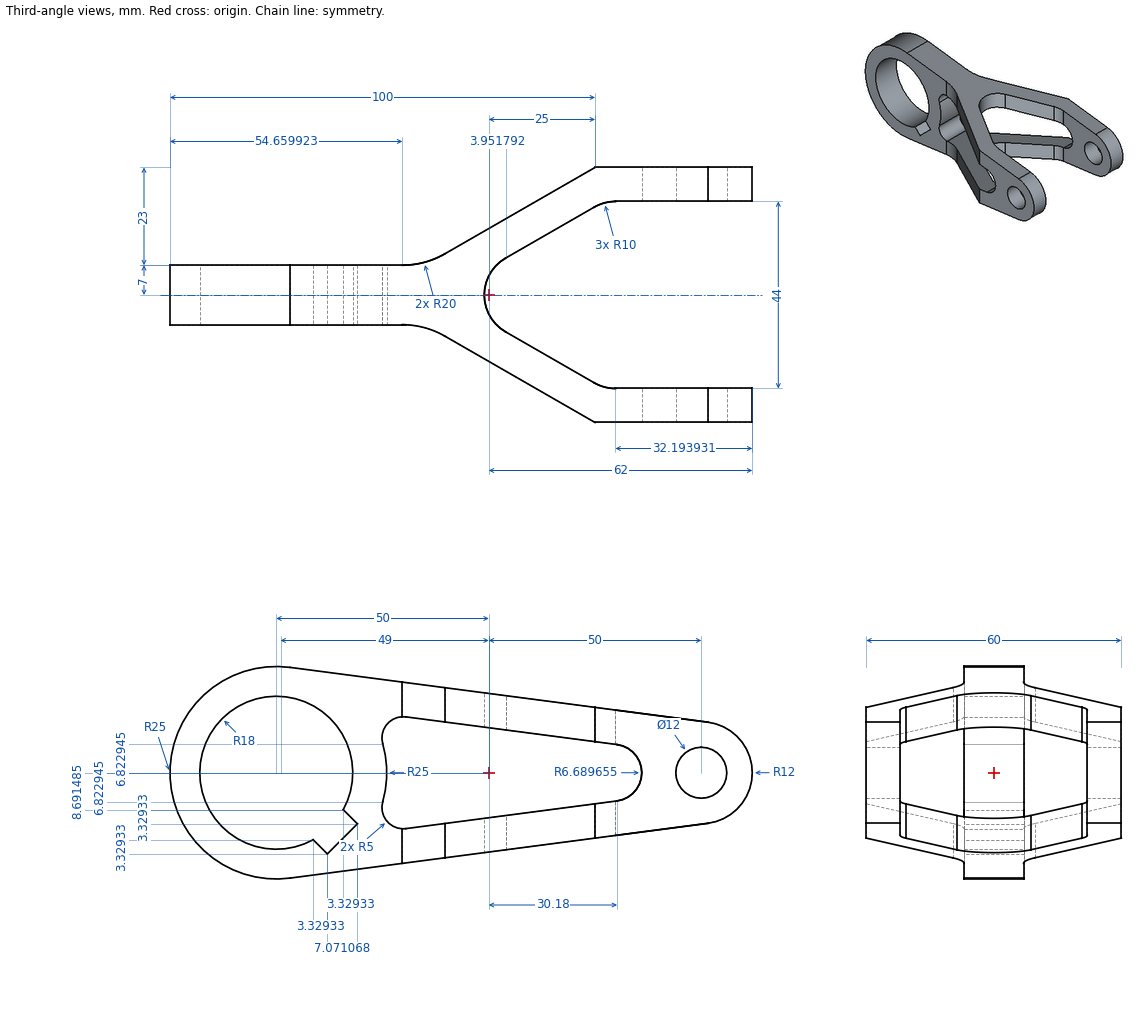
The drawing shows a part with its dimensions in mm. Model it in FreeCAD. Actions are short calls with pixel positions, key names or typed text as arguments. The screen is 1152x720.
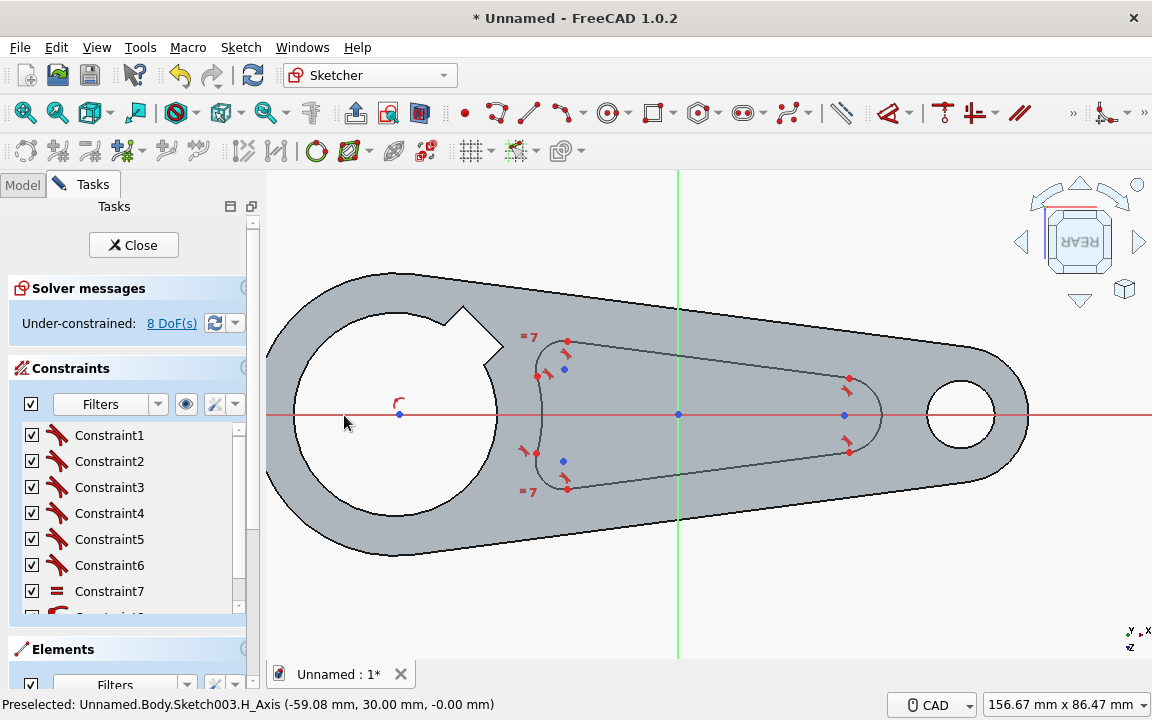
click(844, 415)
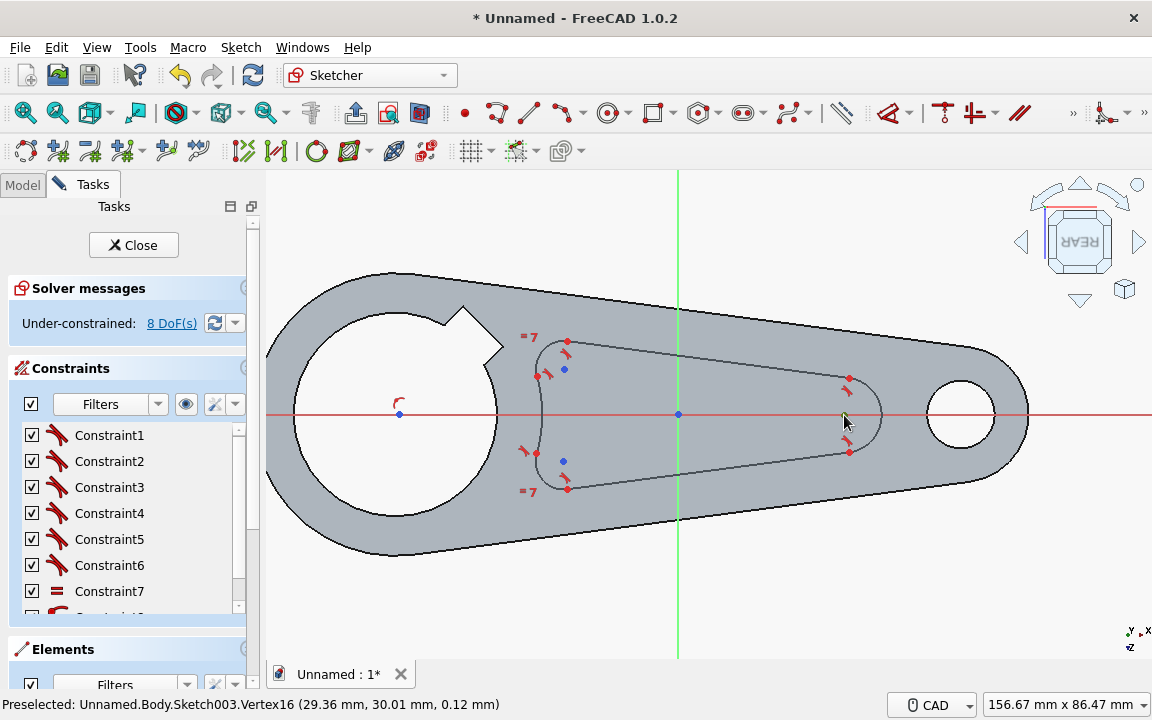
click(344, 415)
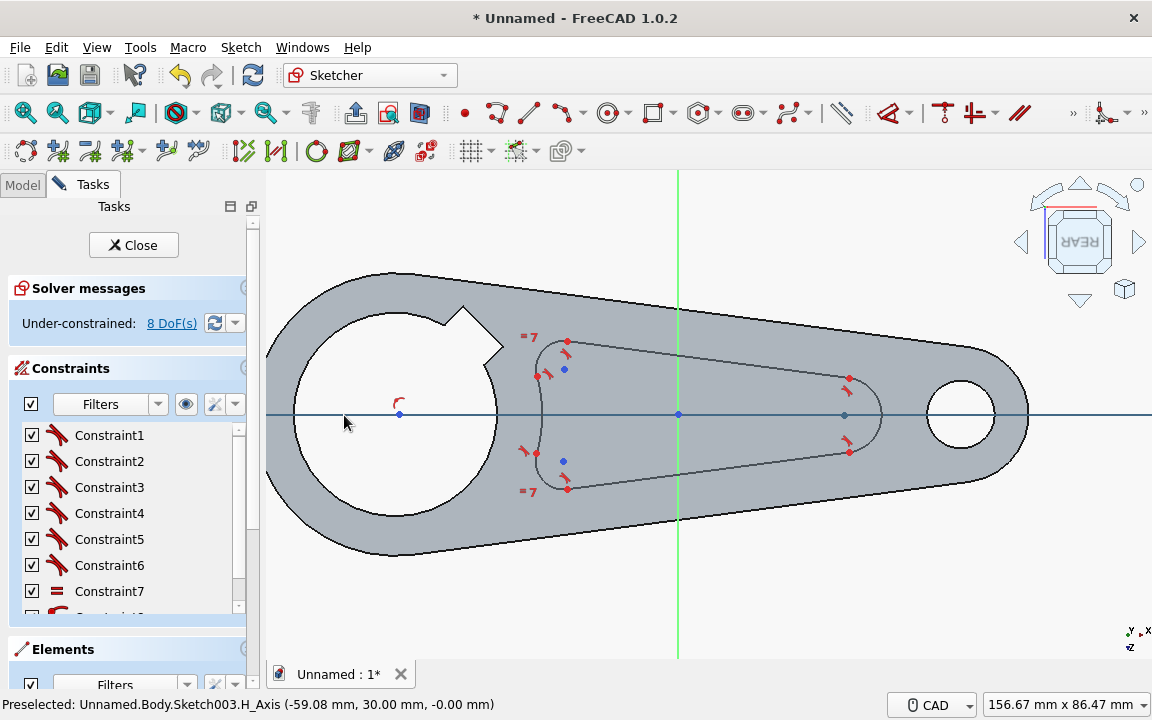
key(c)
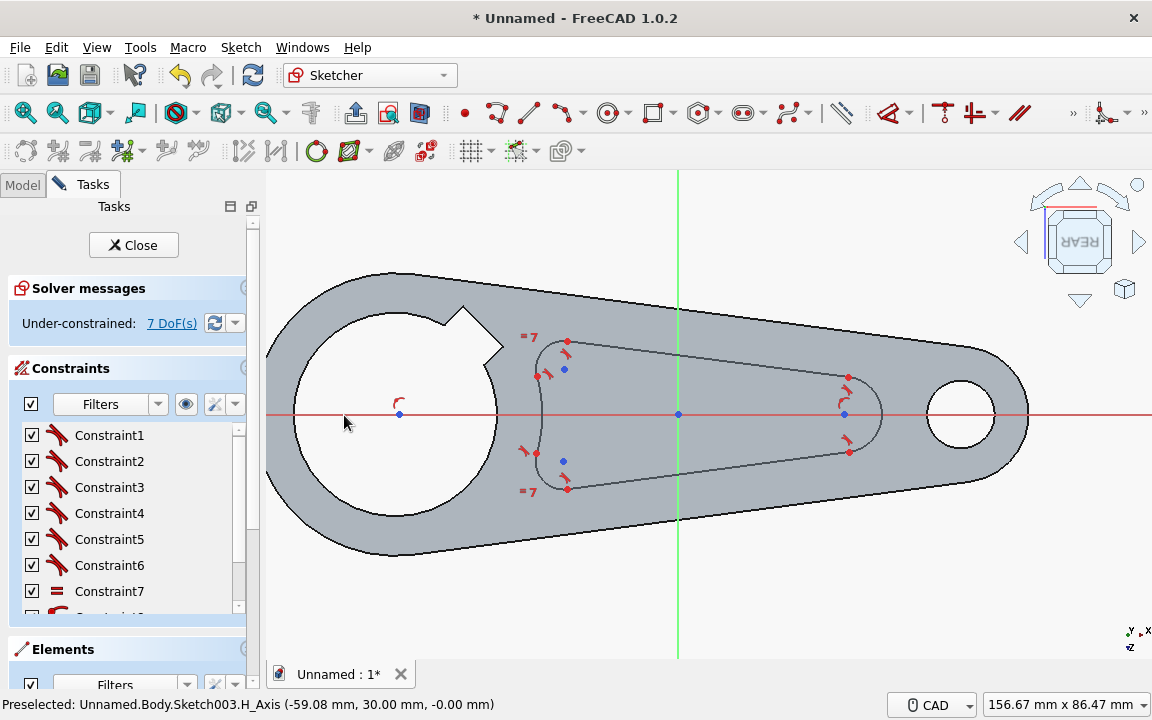
click(888, 114)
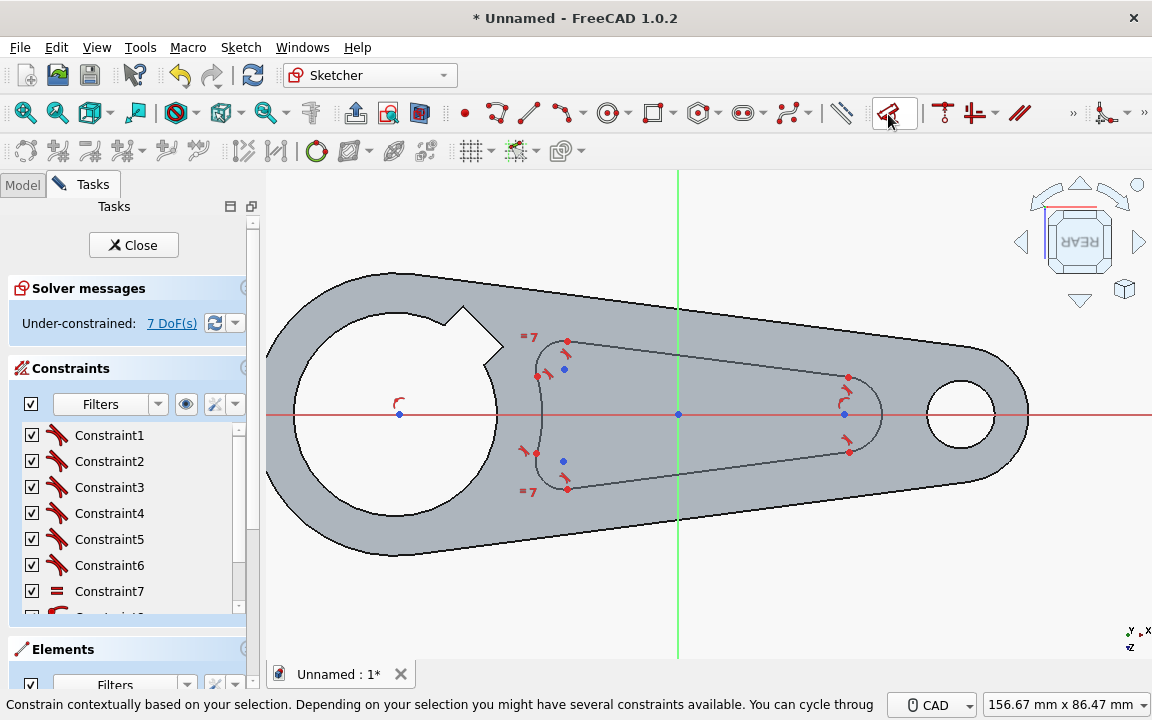
scroll(552, 344, up, 2)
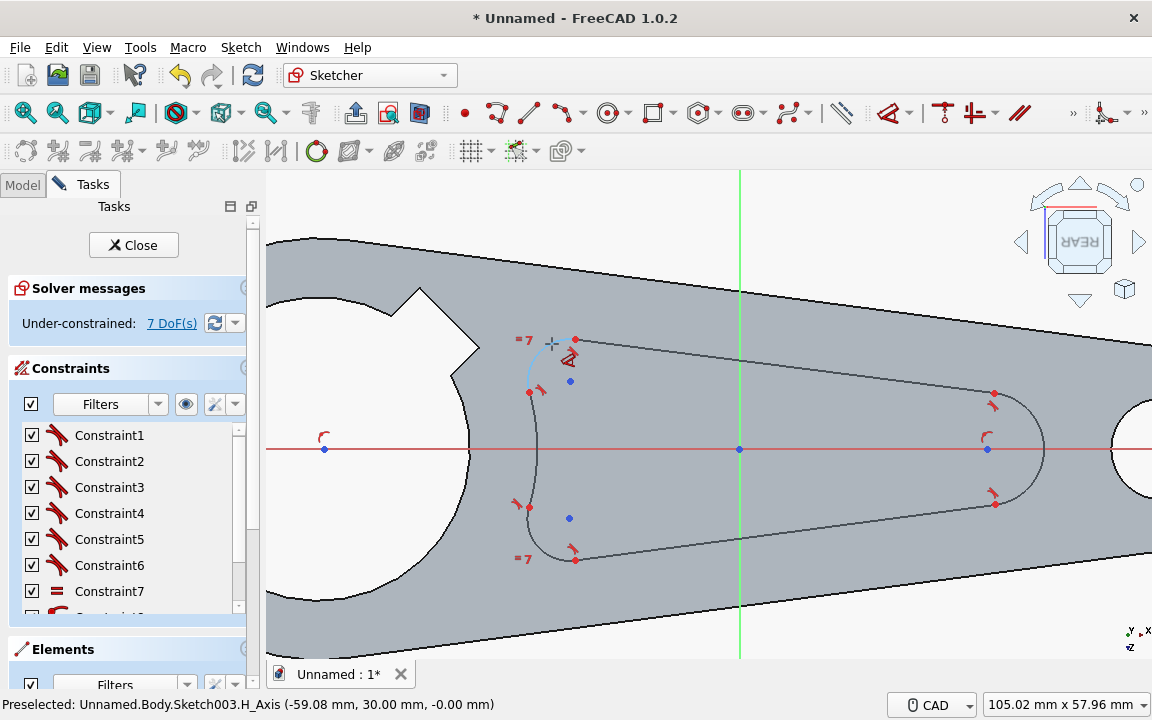
click(551, 344)
click(536, 316)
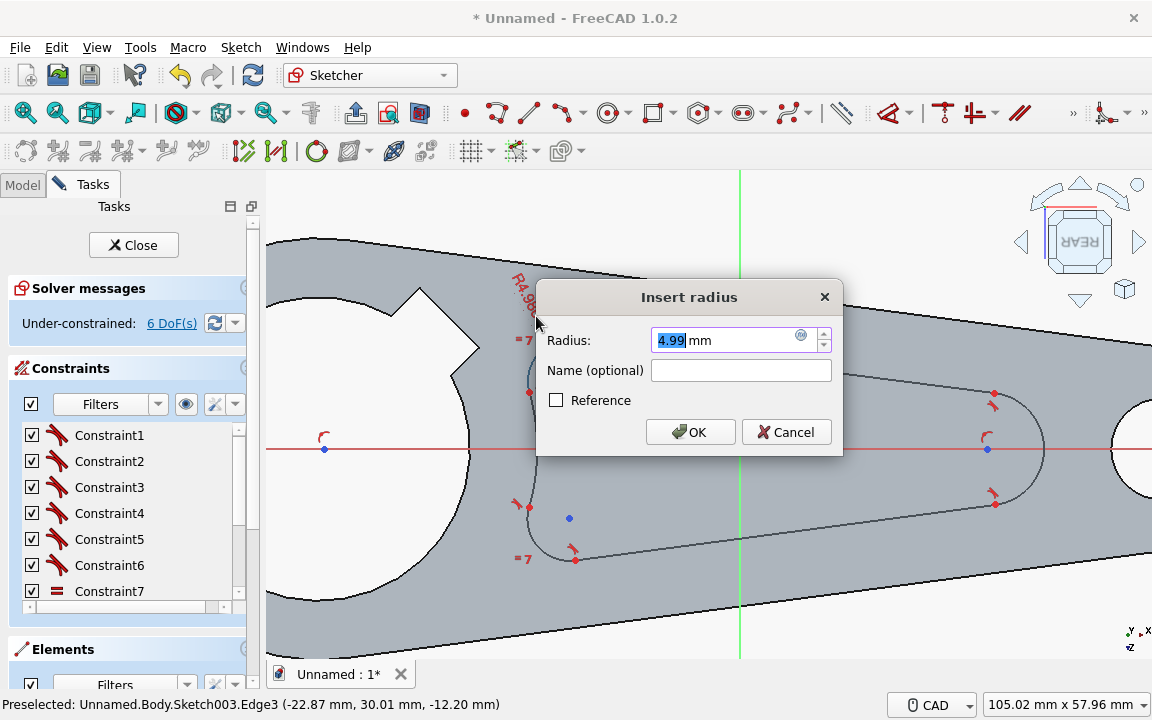
text(5)
key(Return)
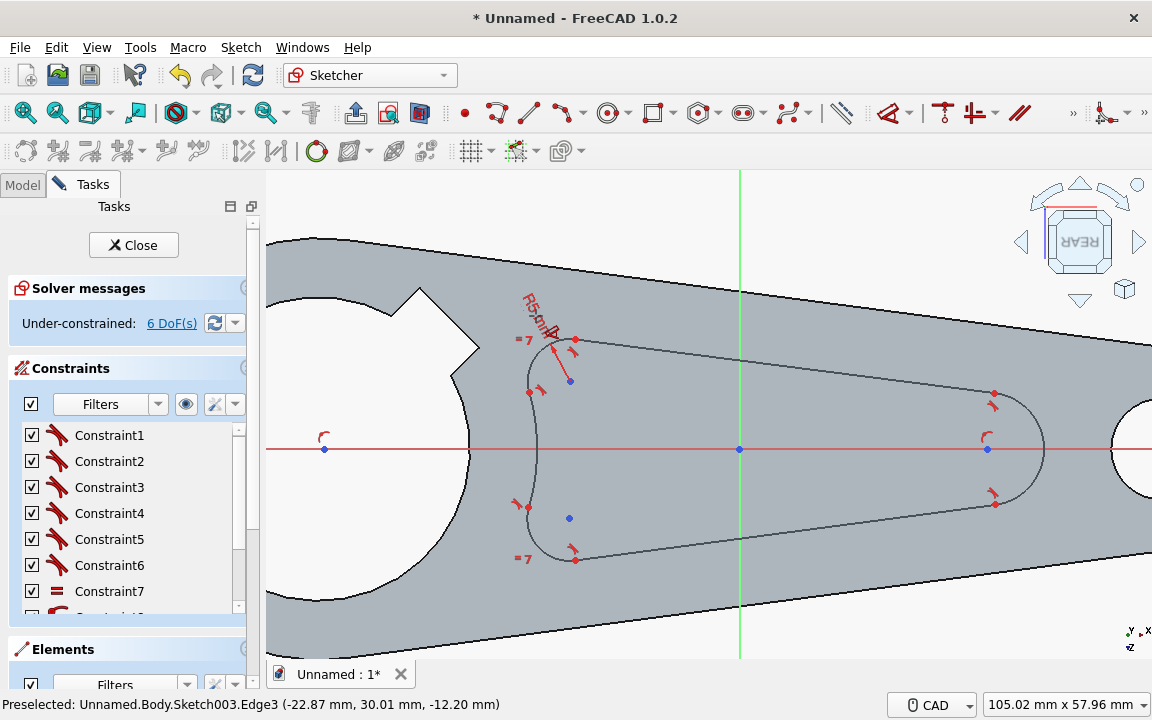
click(536, 473)
click(568, 477)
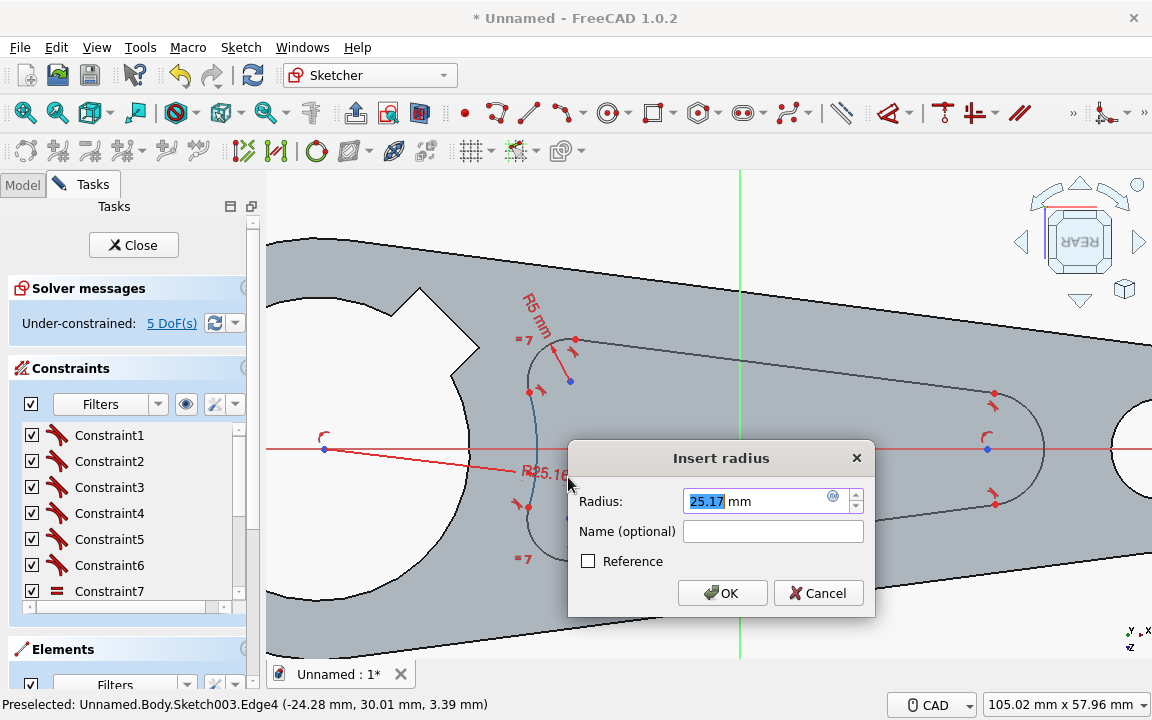
text(25)
key(Return)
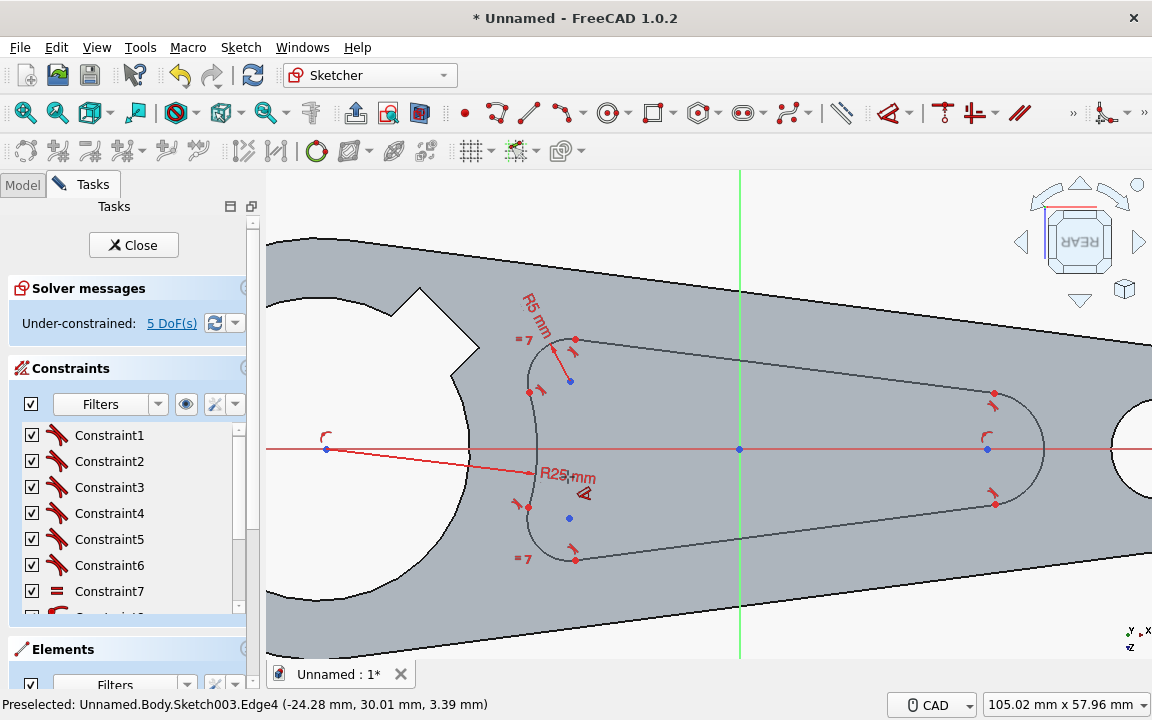
scroll(294, 258, down, 1)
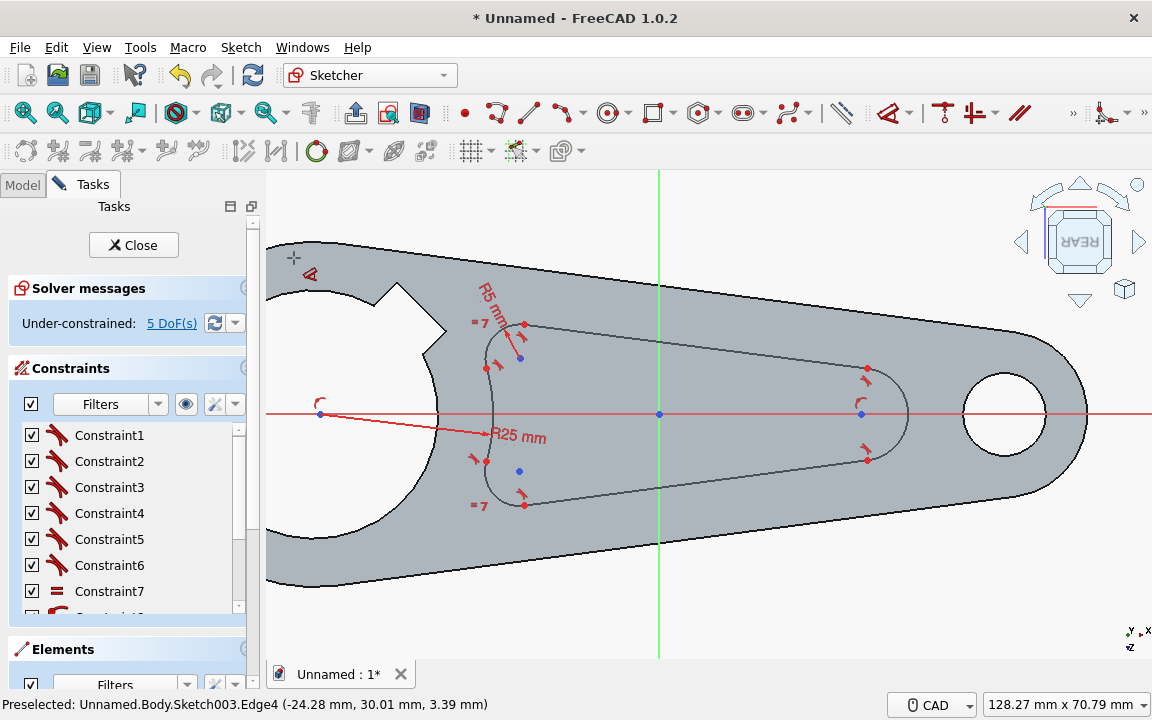
click(901, 440)
click(928, 458)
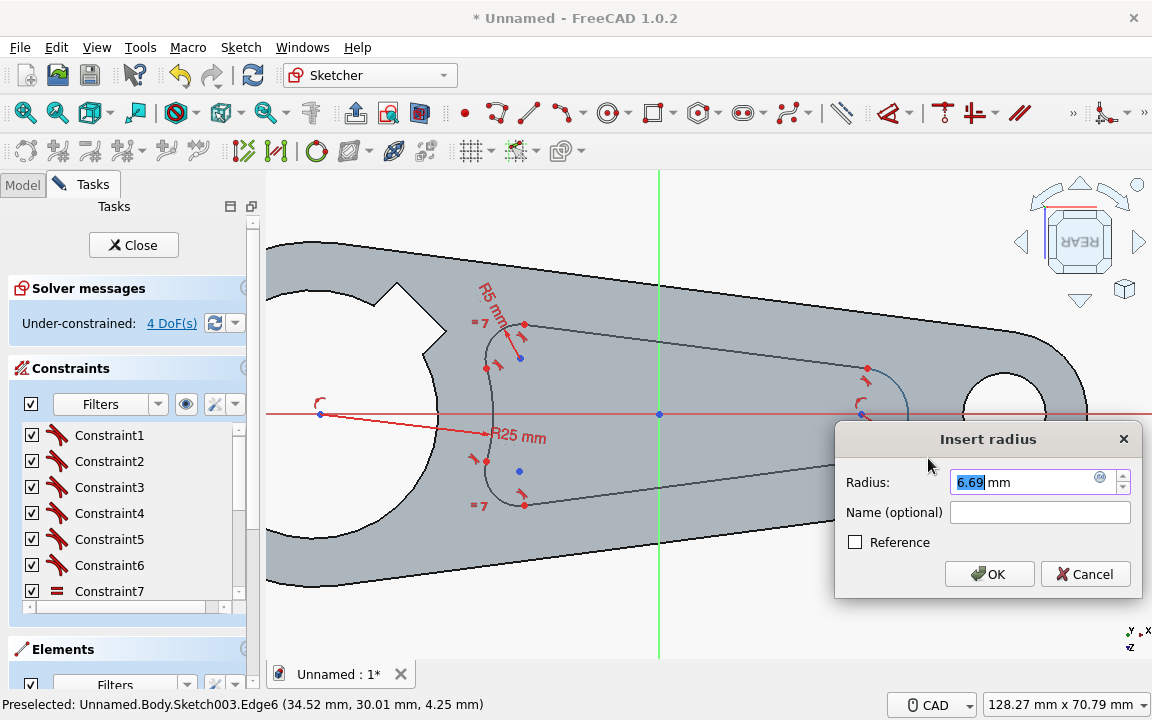
text(6.689655)
key(Return)